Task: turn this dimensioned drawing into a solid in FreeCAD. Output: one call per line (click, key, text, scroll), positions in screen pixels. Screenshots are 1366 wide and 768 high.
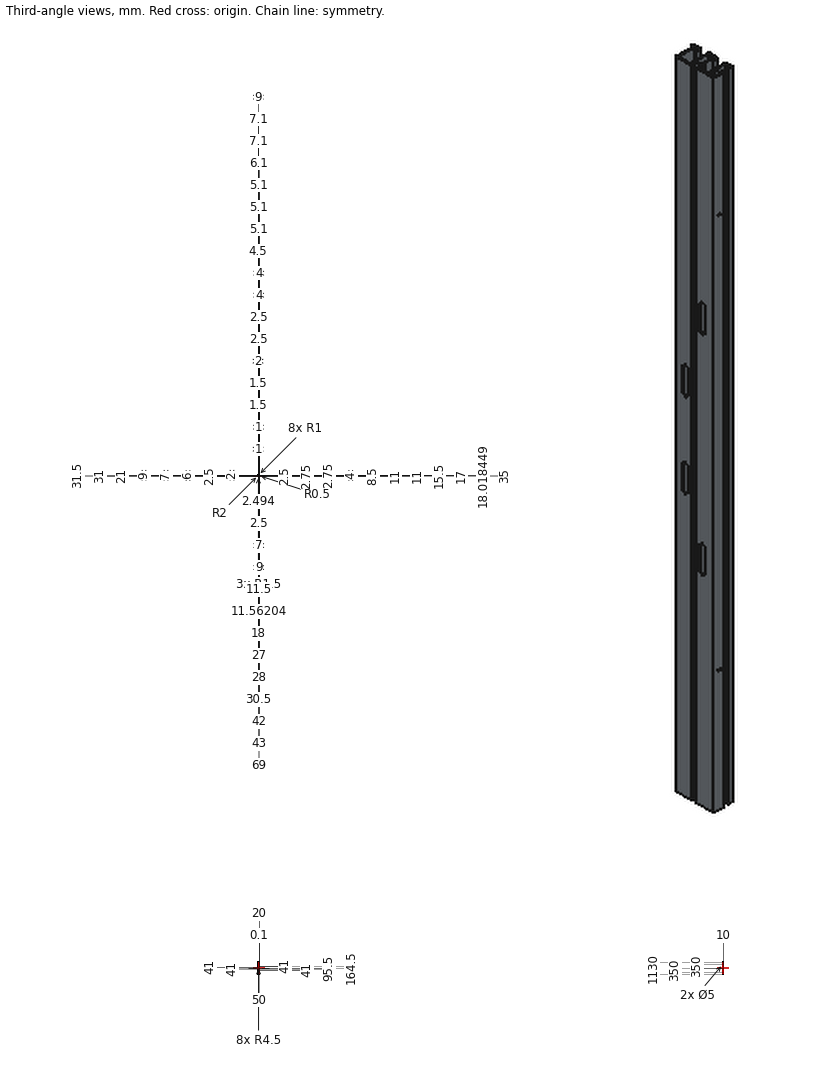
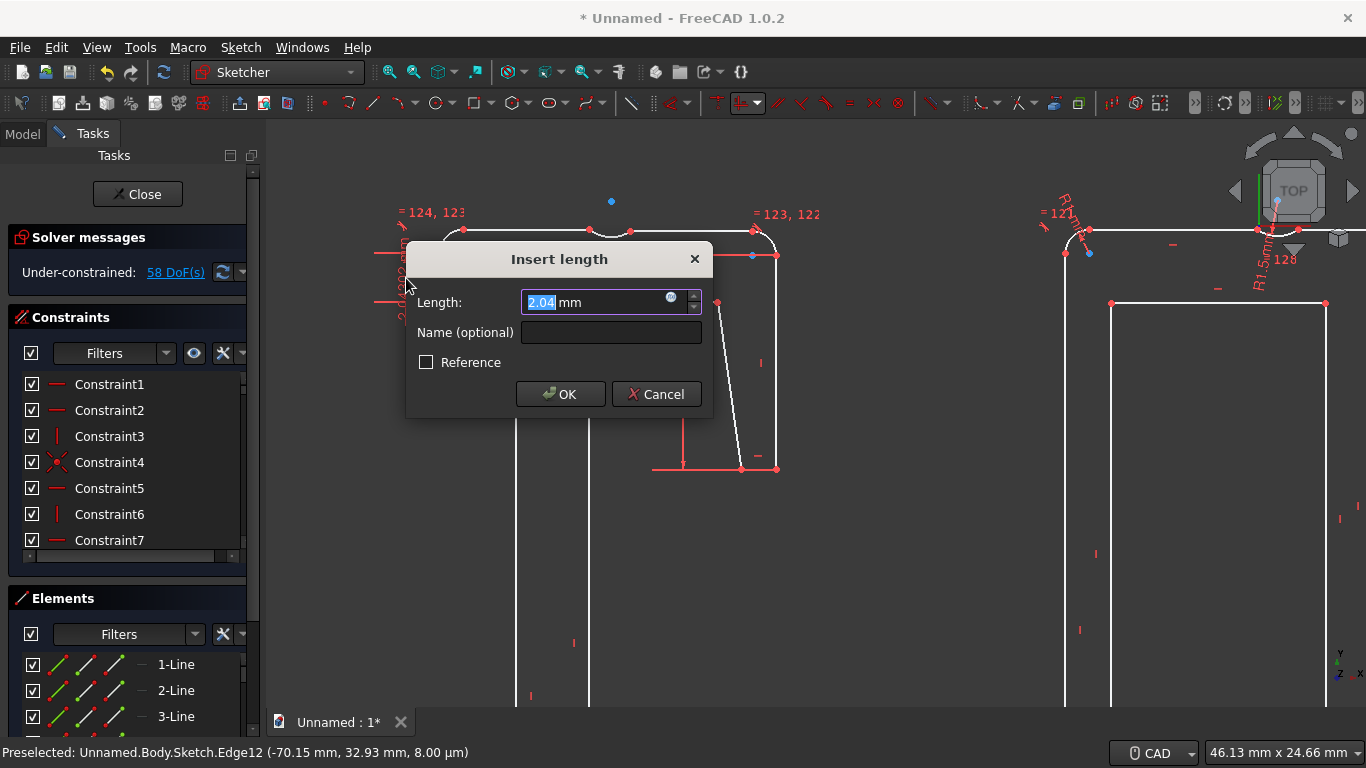
text(2)
key(Return)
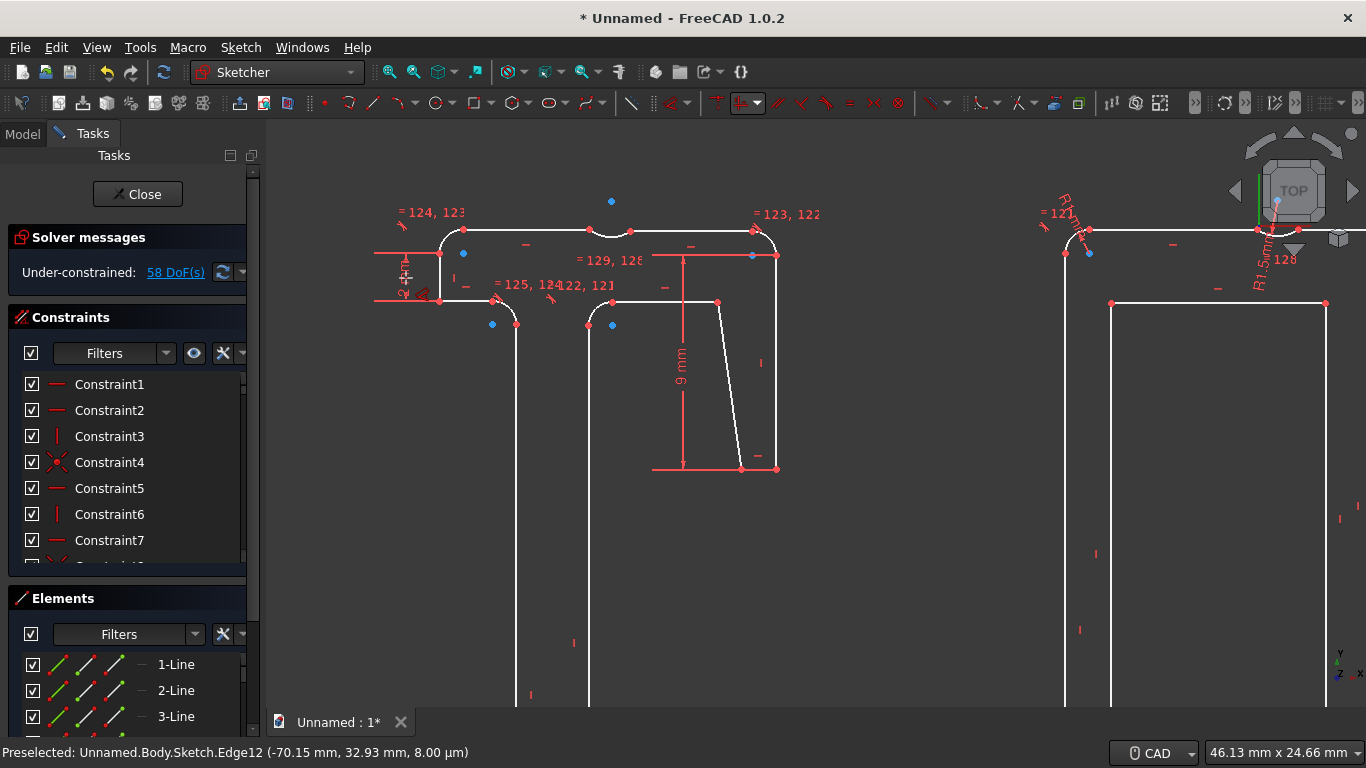
click(456, 301)
click(478, 267)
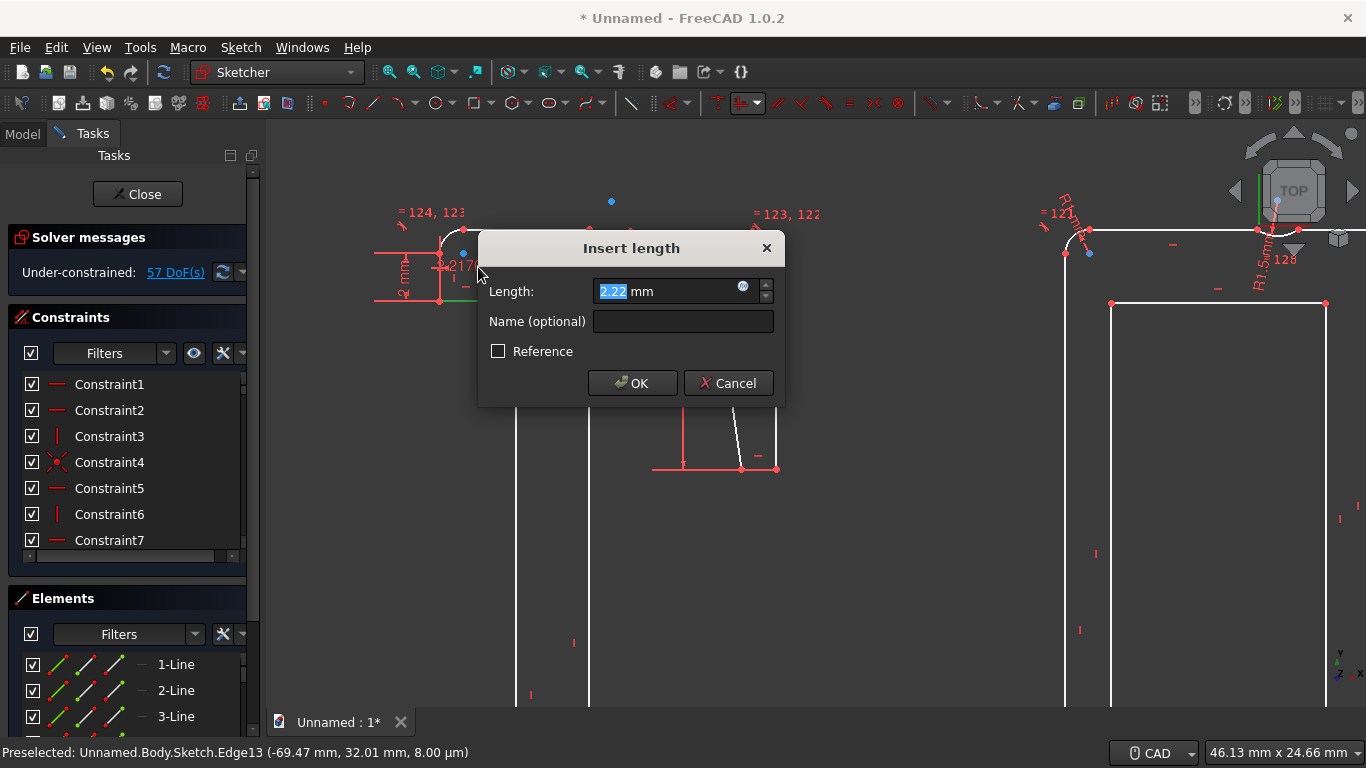
text(2)
key(Return)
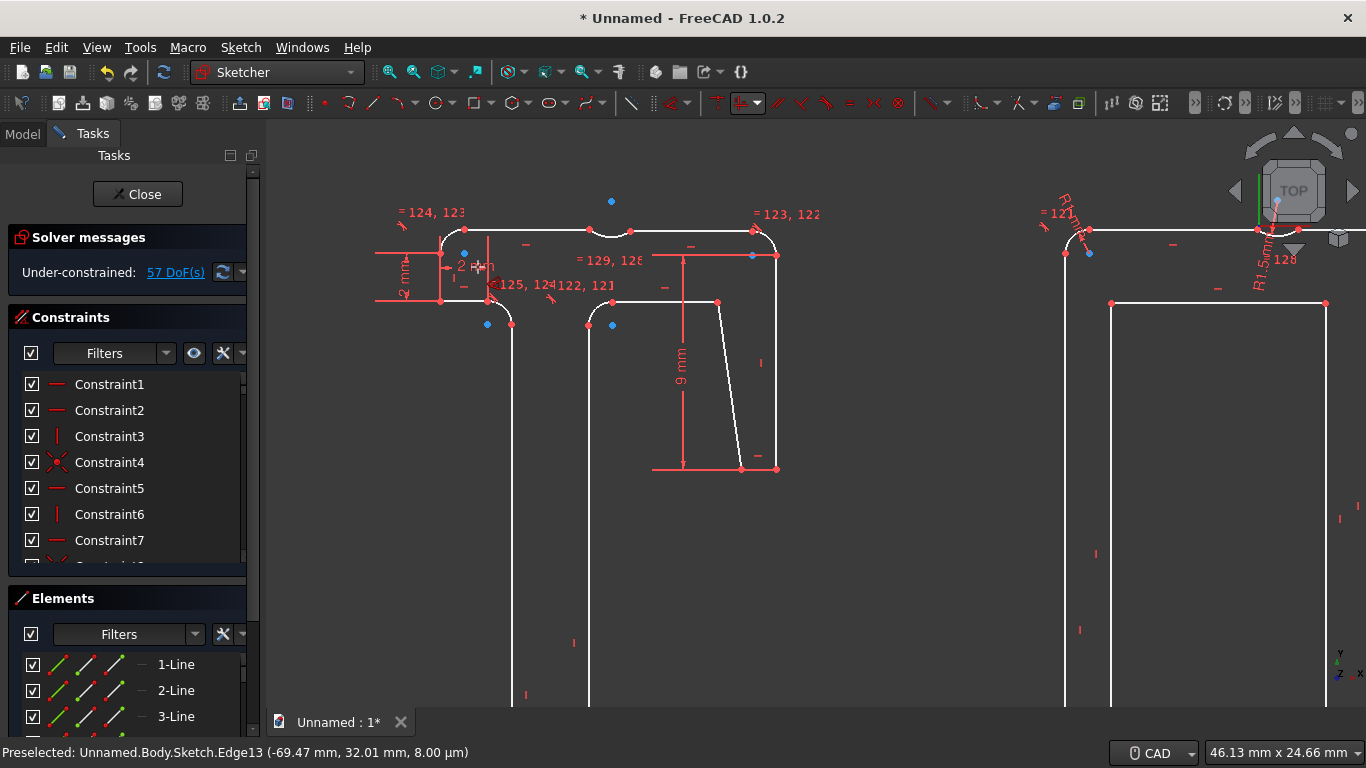
scroll(439, 277, down, 5)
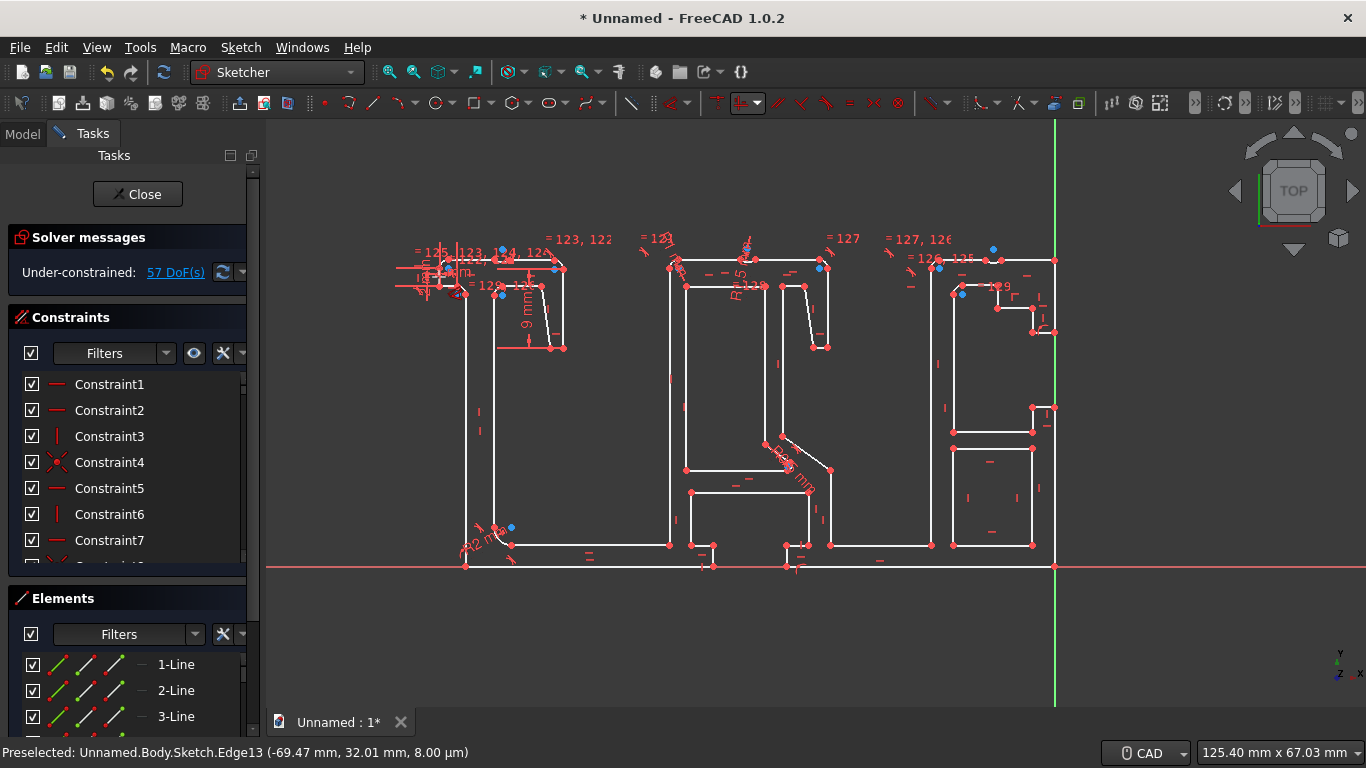
click(691, 530)
click(725, 519)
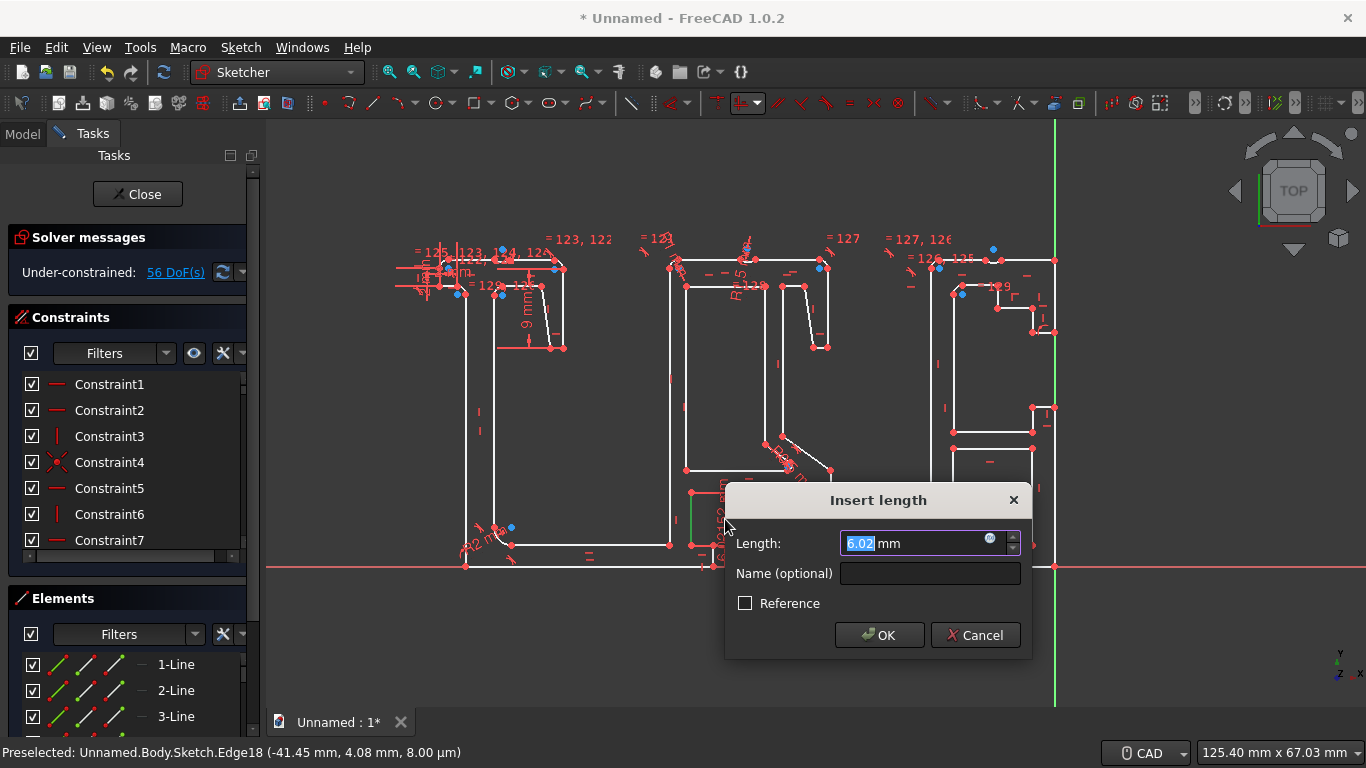
text(6)
key(Return)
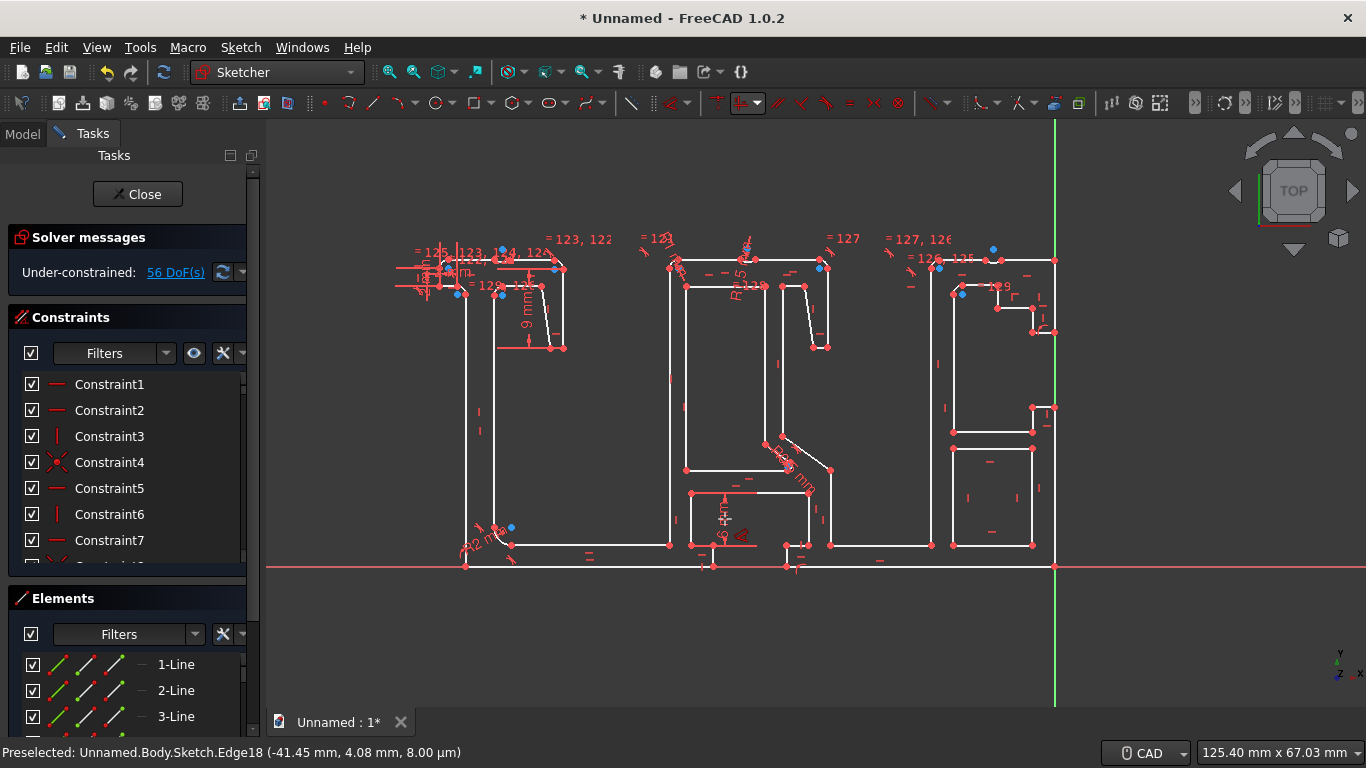
click(809, 509)
click(867, 519)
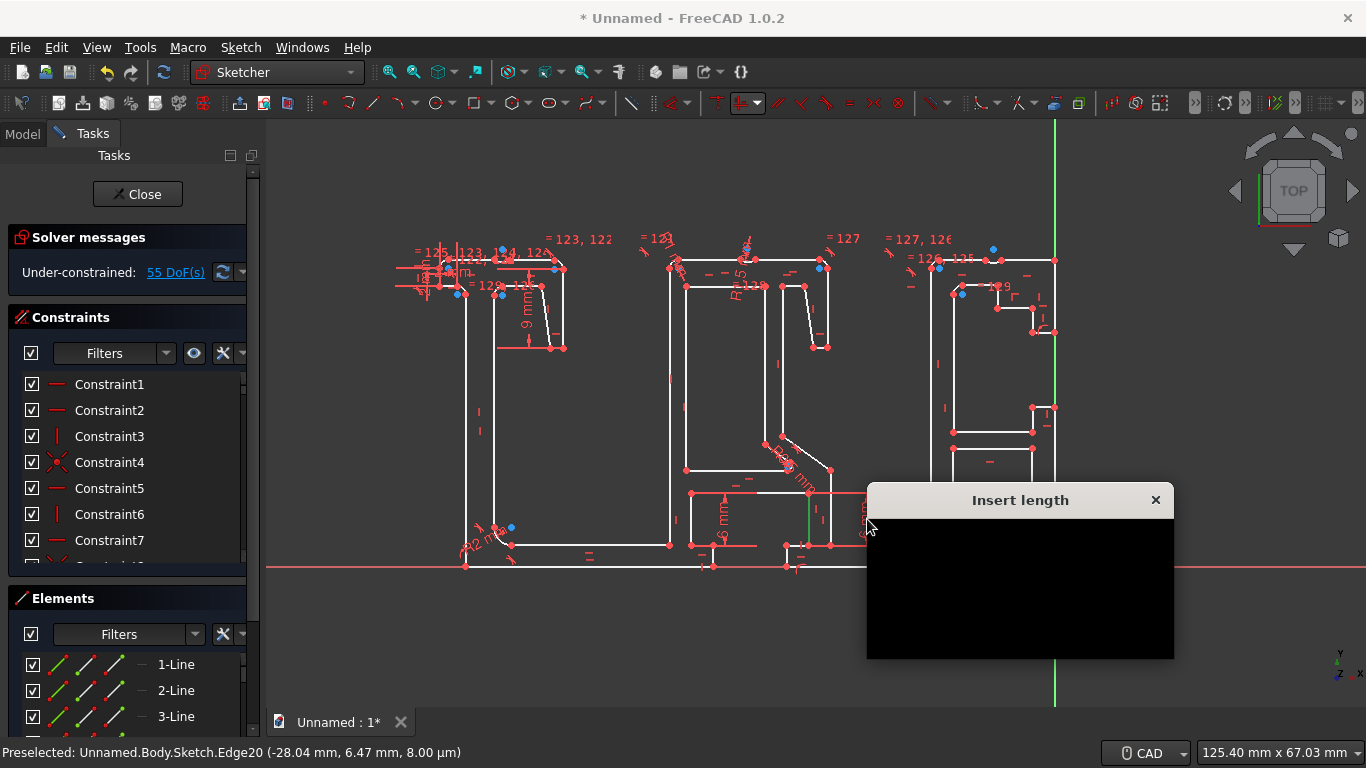
text(6)
key(Return)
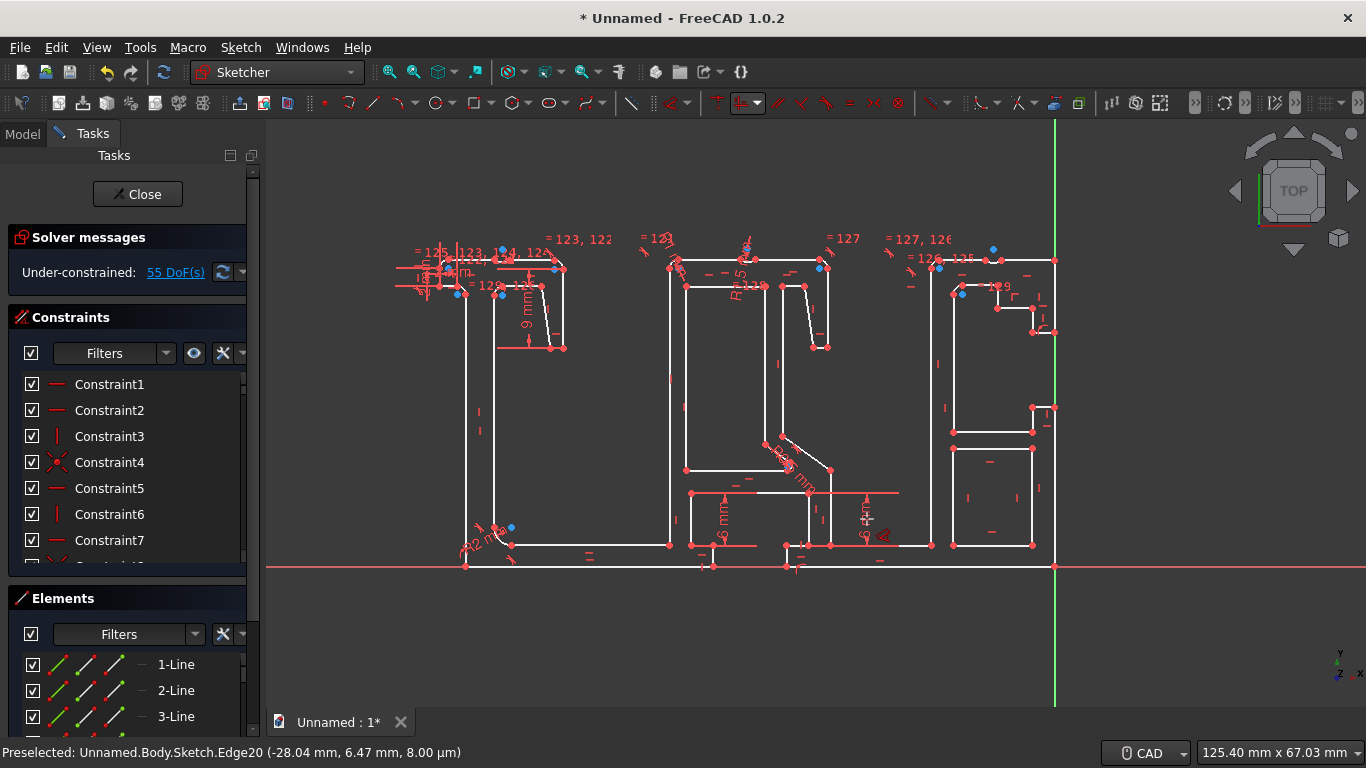
click(1009, 432)
click(993, 466)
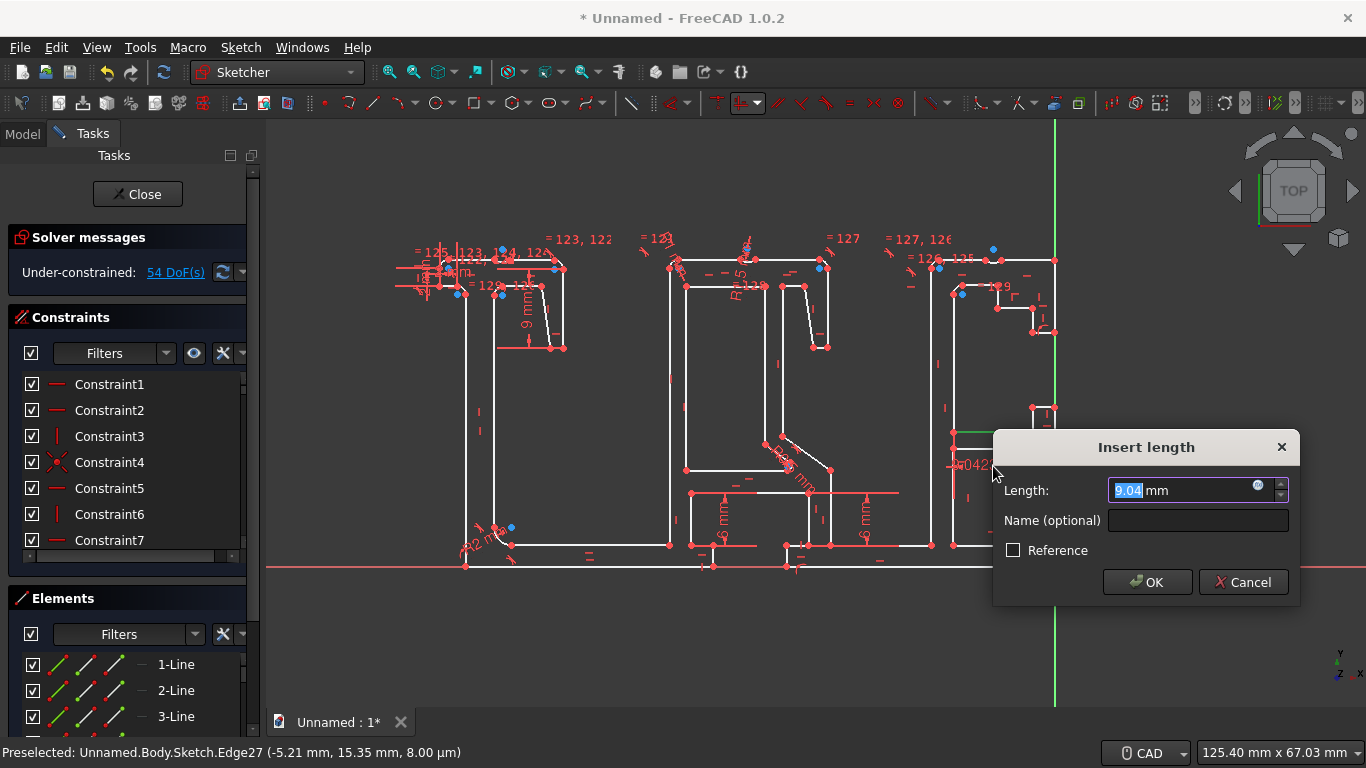
text(9)
key(Return)